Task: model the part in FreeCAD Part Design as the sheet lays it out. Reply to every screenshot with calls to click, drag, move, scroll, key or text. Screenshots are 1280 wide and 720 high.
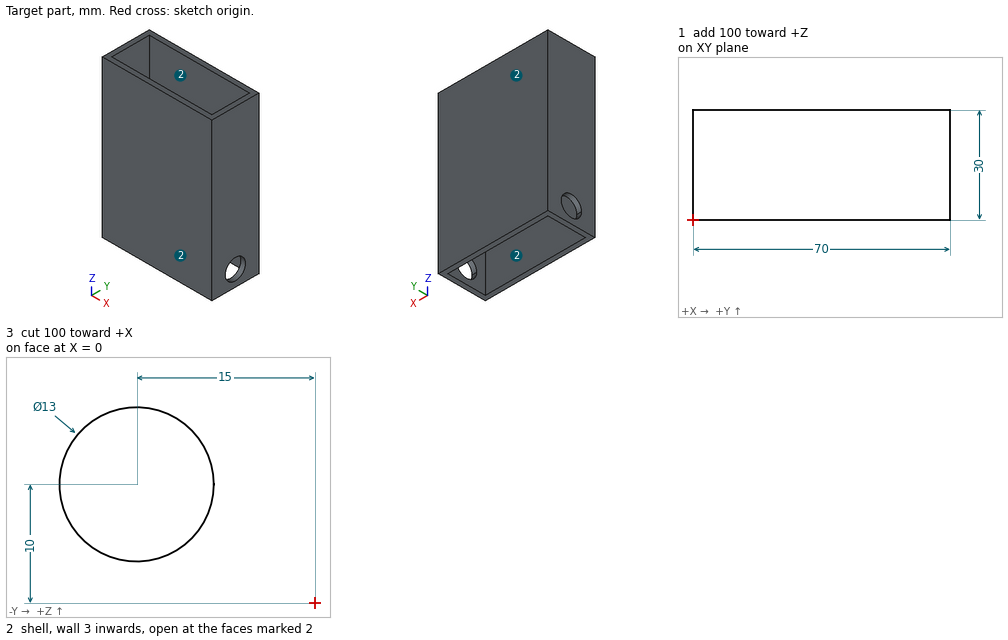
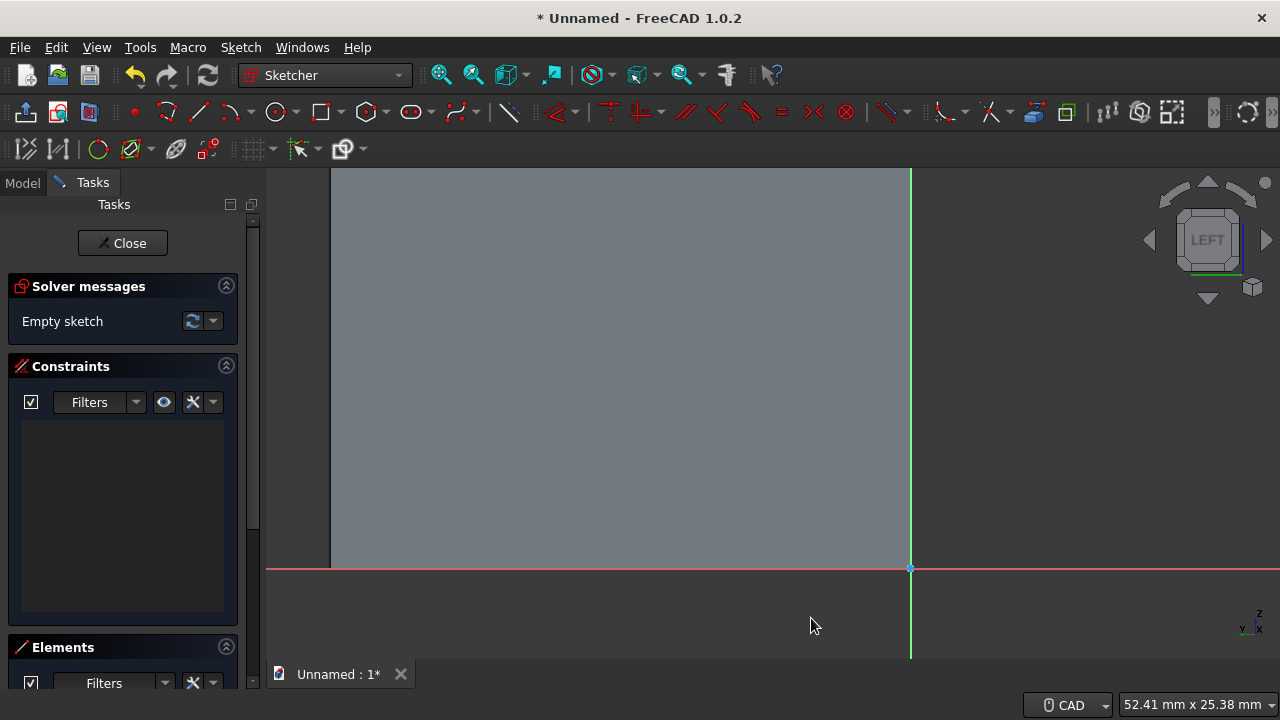
click(276, 112)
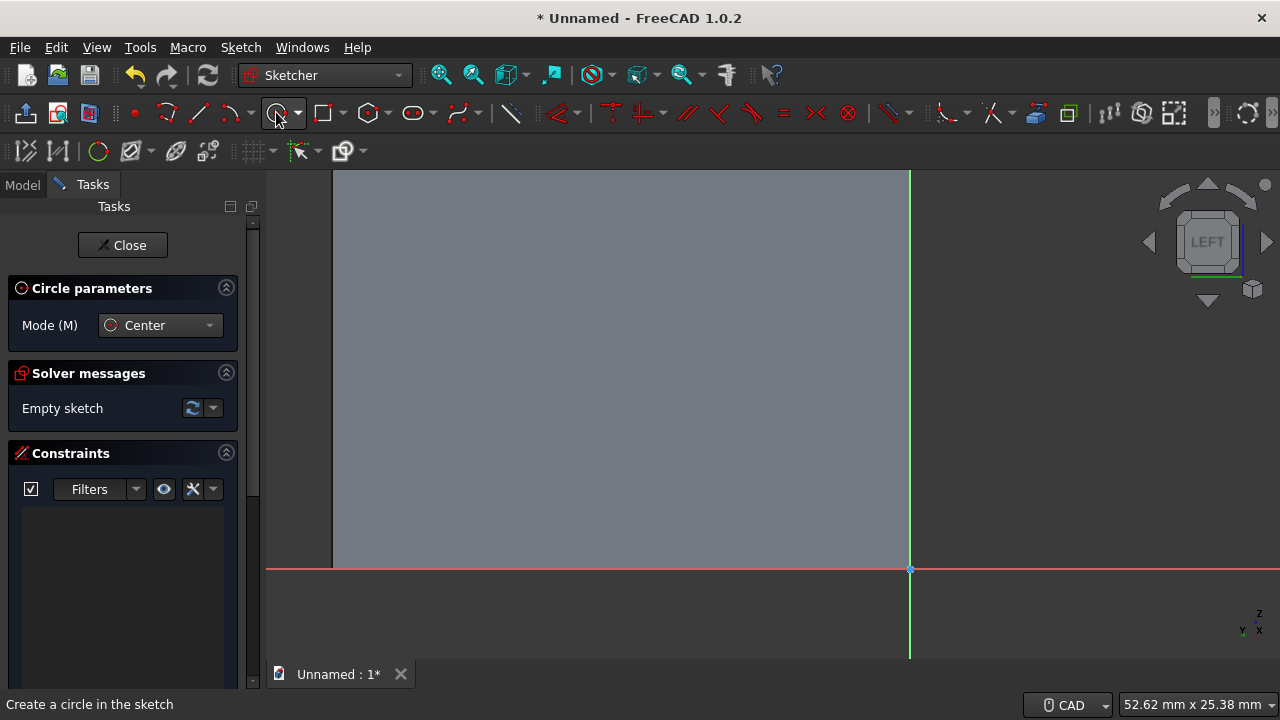
click(621, 377)
move(710, 288)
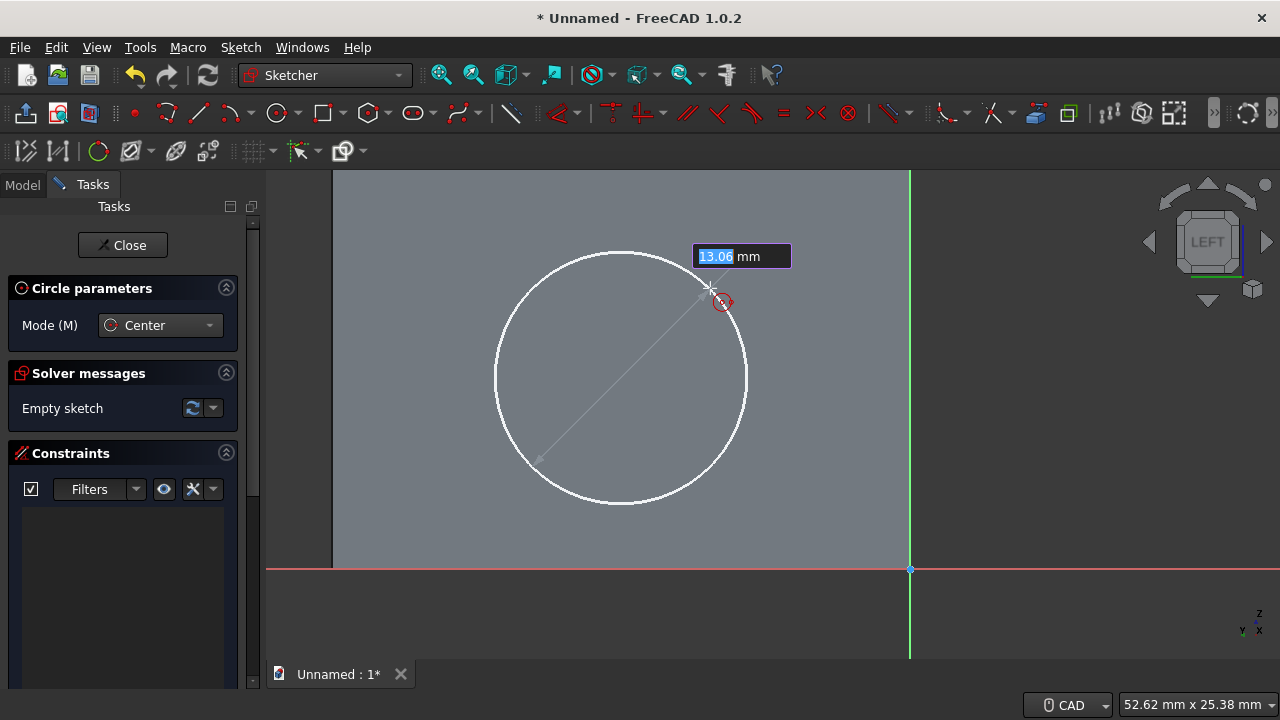
text(13)
key(Return)
key(Escape)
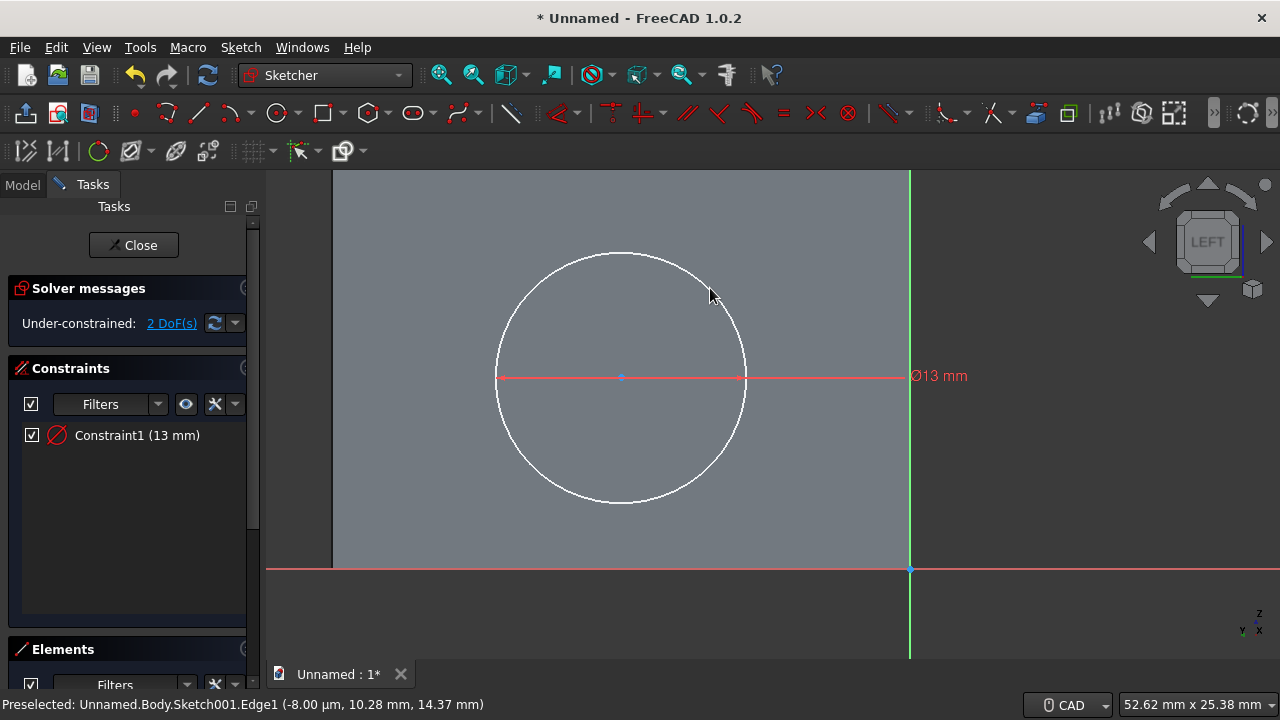
click(558, 114)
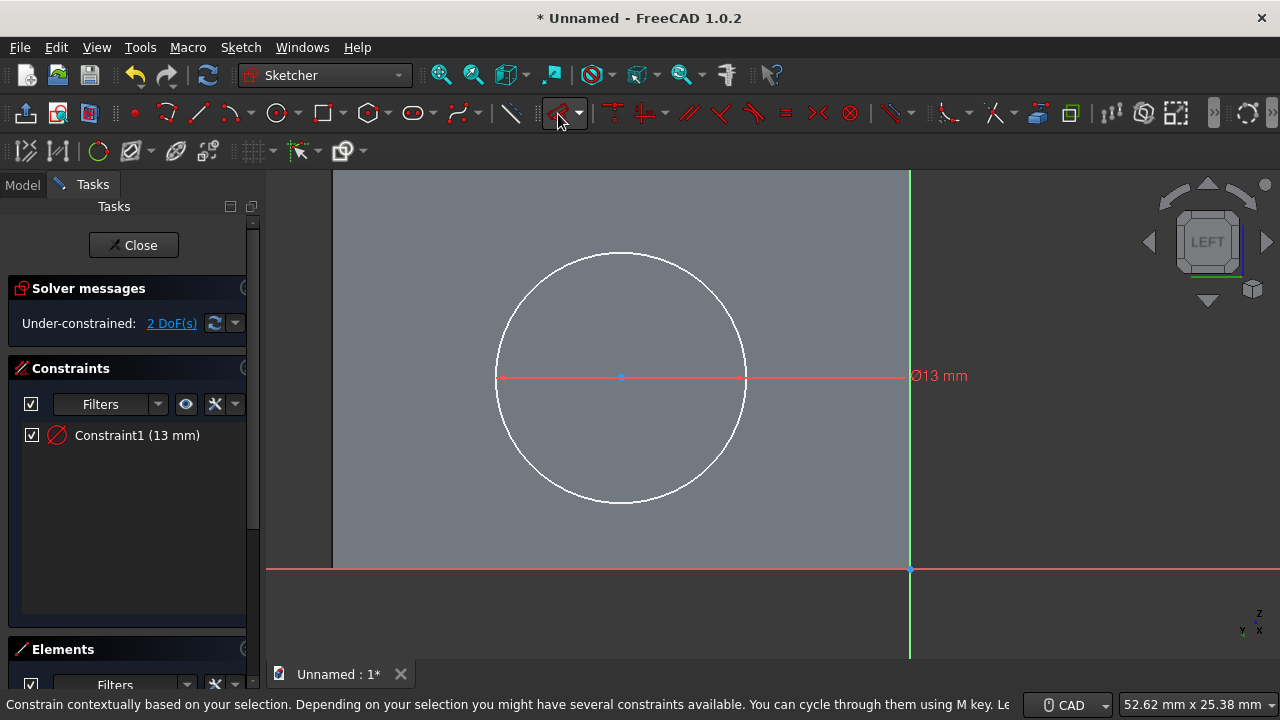
click(621, 378)
click(766, 603)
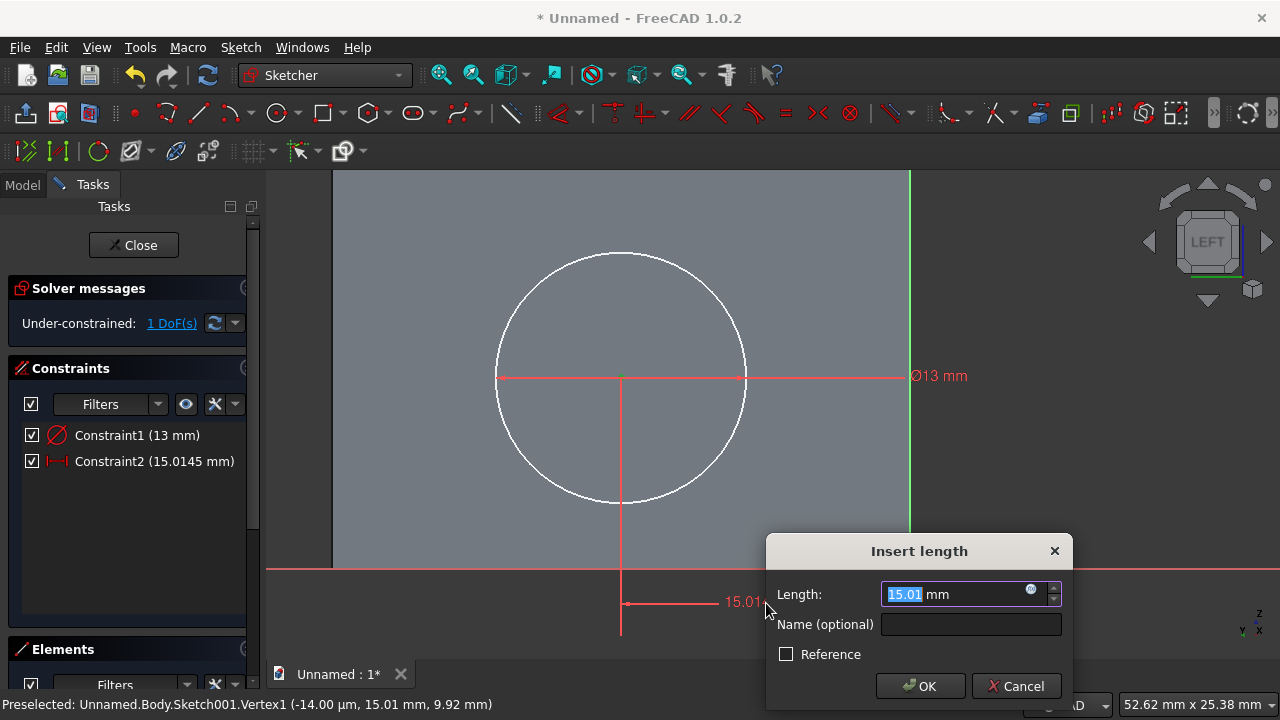
text(15)
key(Return)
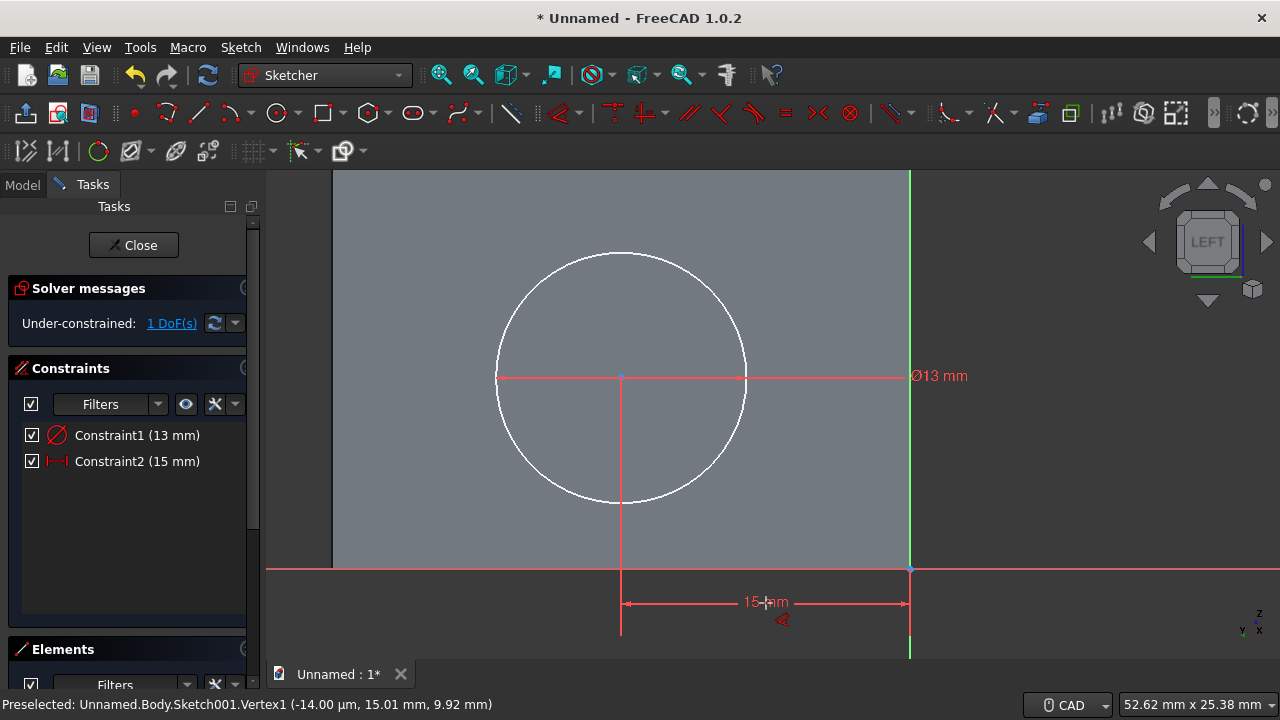
click(621, 378)
click(944, 474)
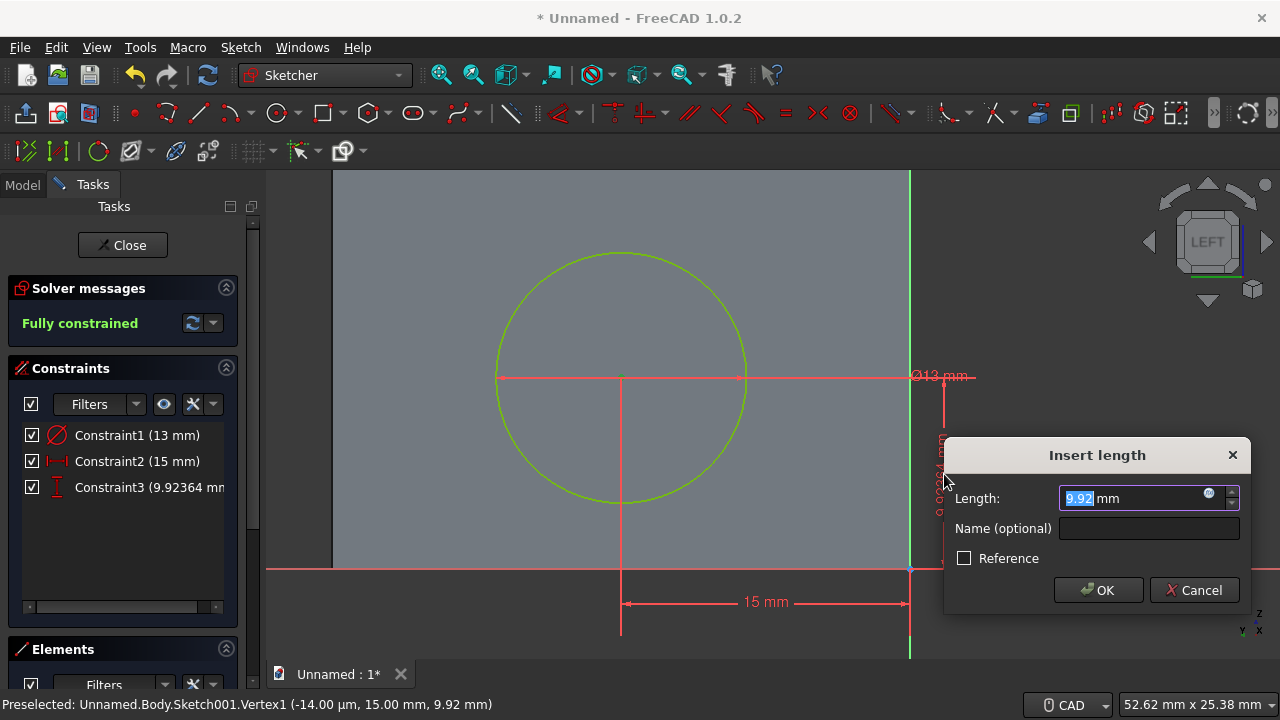
text(10)
key(Return)
key(Escape)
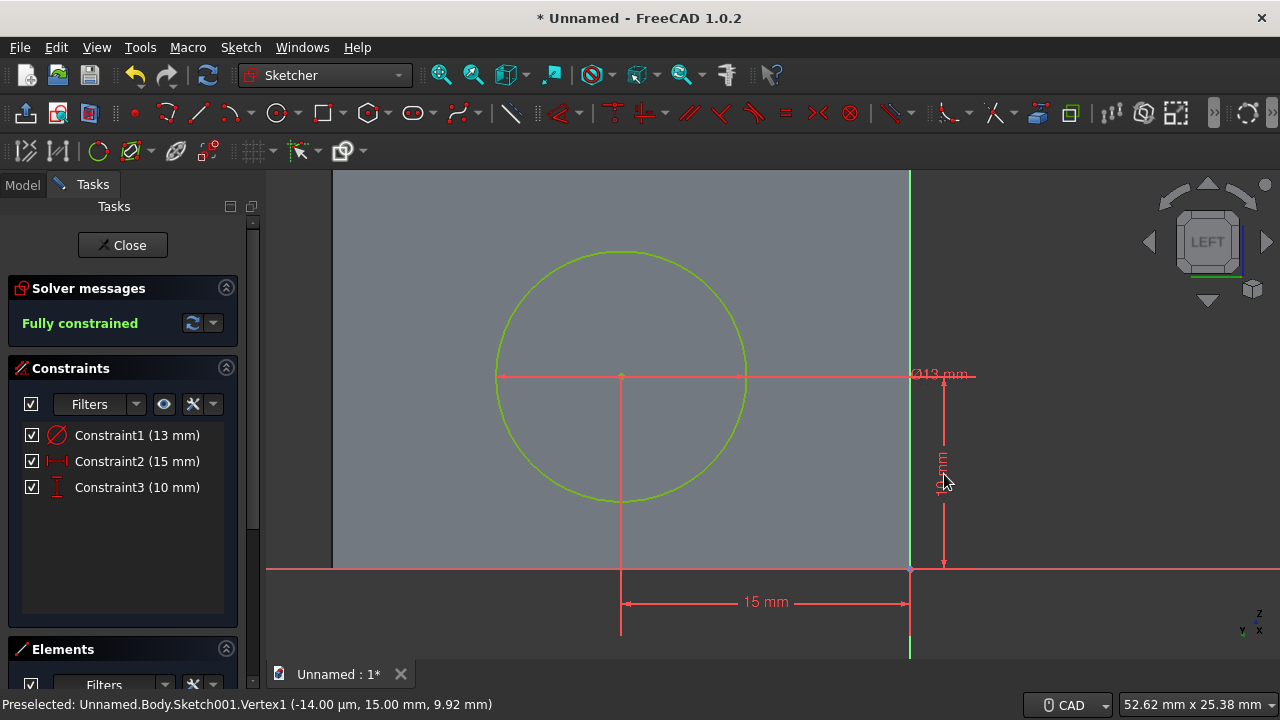
click(123, 245)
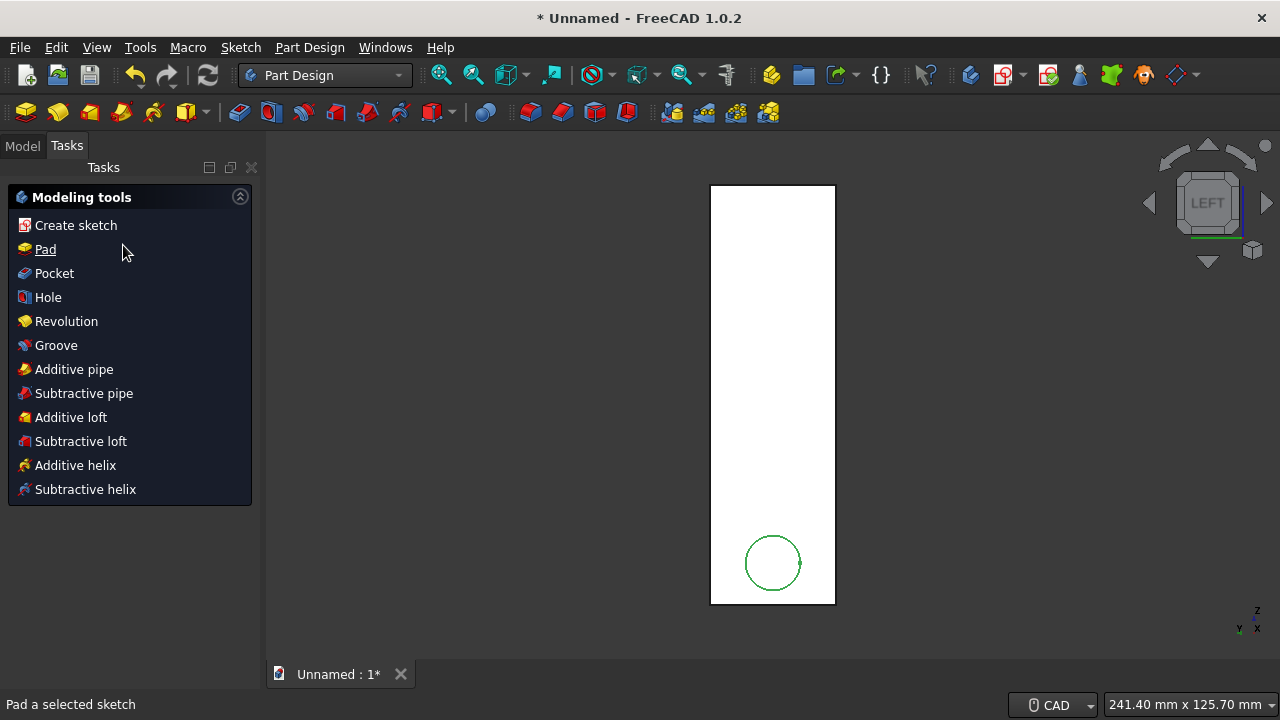
click(240, 112)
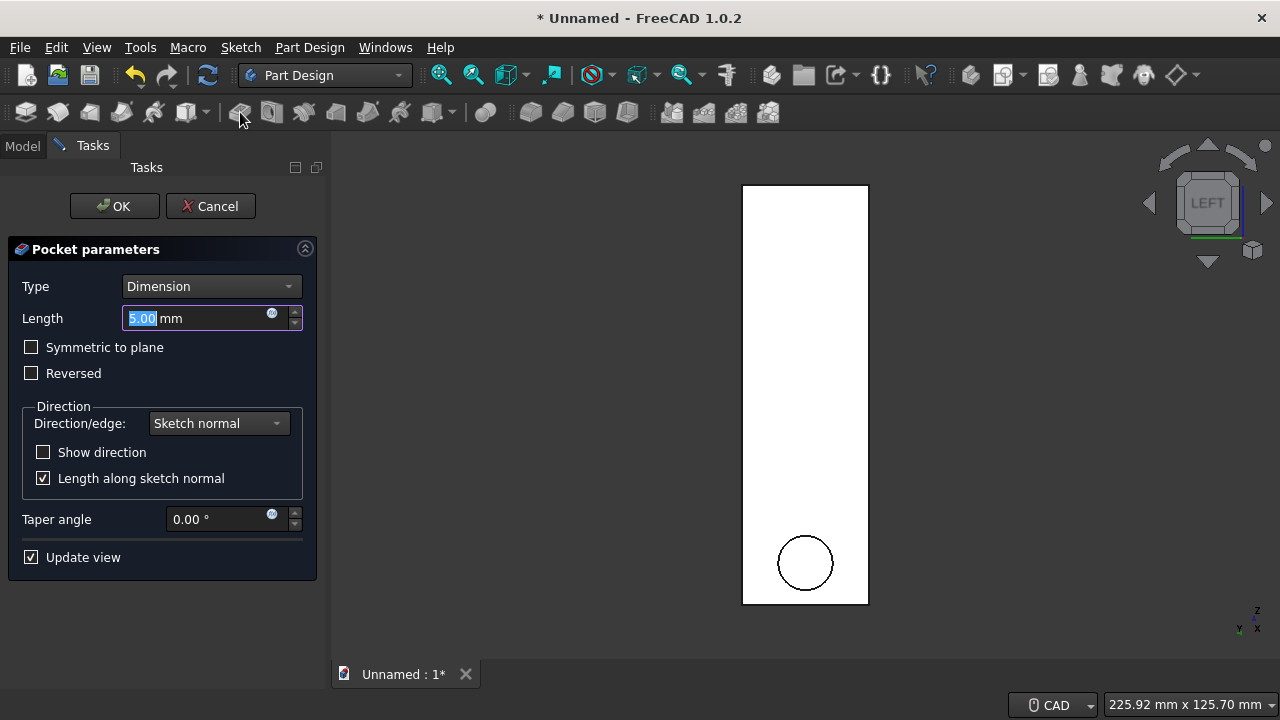
text(100)
key(Tab)